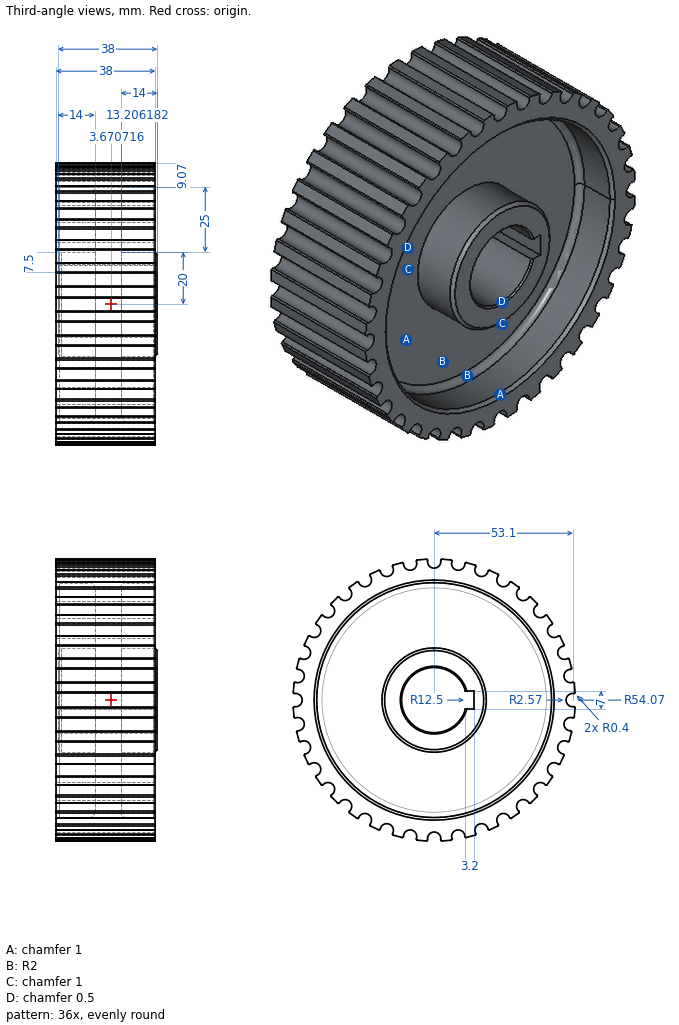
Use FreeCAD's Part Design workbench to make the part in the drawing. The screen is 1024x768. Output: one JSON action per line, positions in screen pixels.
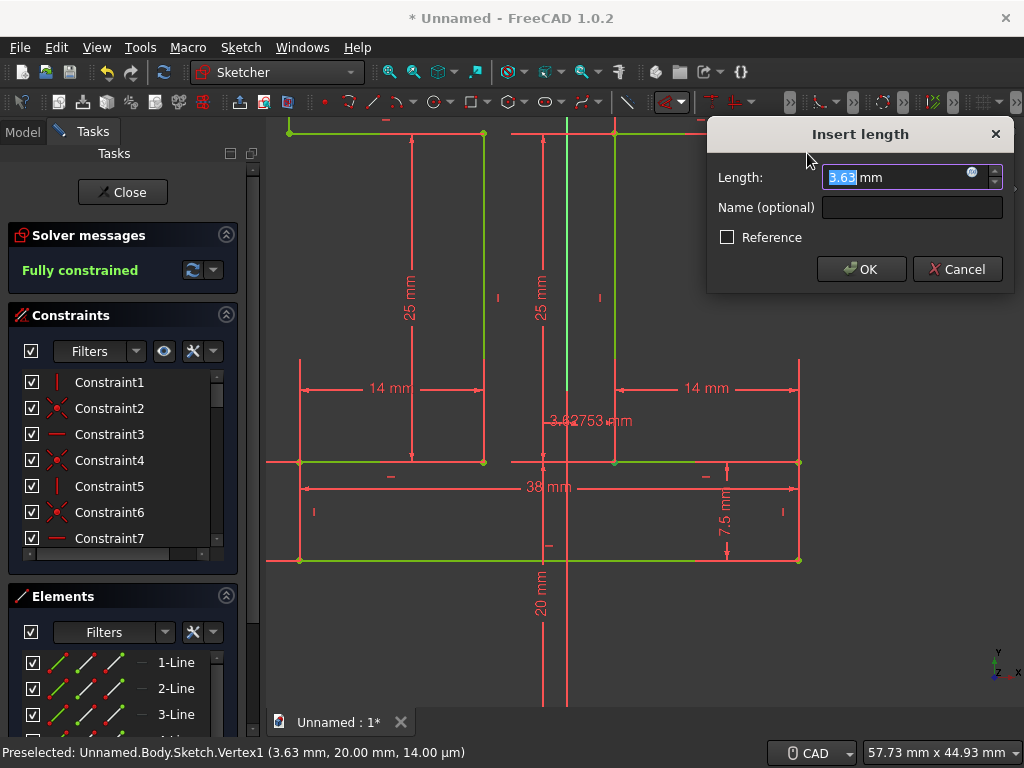
{"action": "type", "text": "3.670716"}
{"action": "key", "text": "Return"}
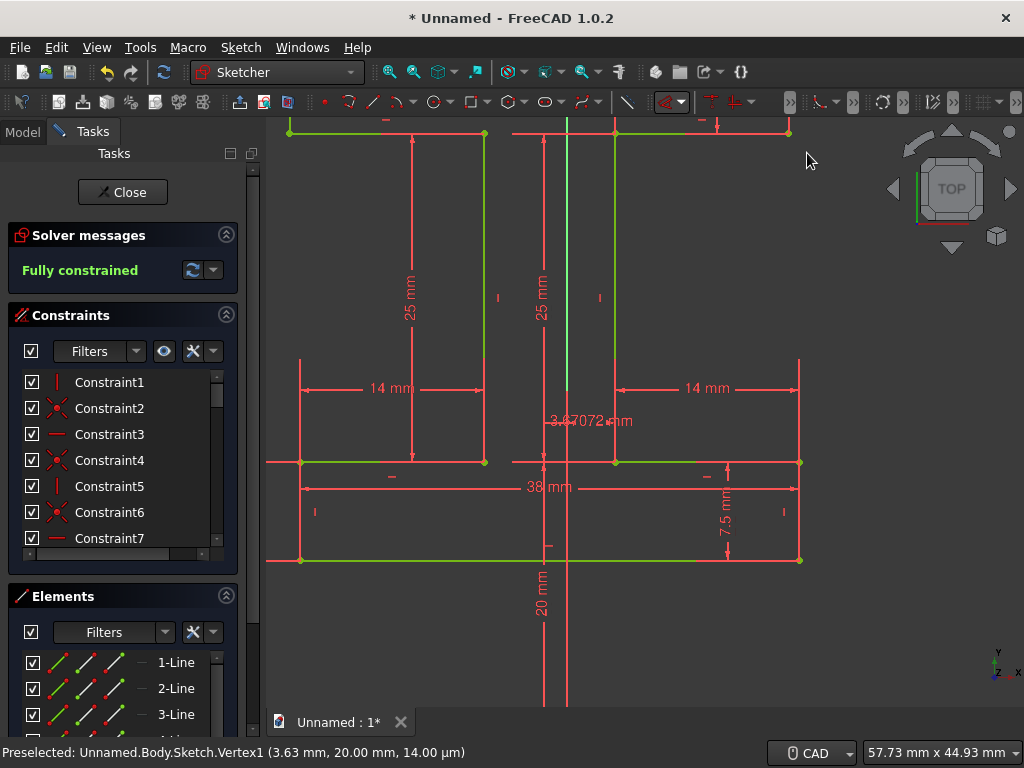
{"action": "left_click", "coordinate": [123, 192]}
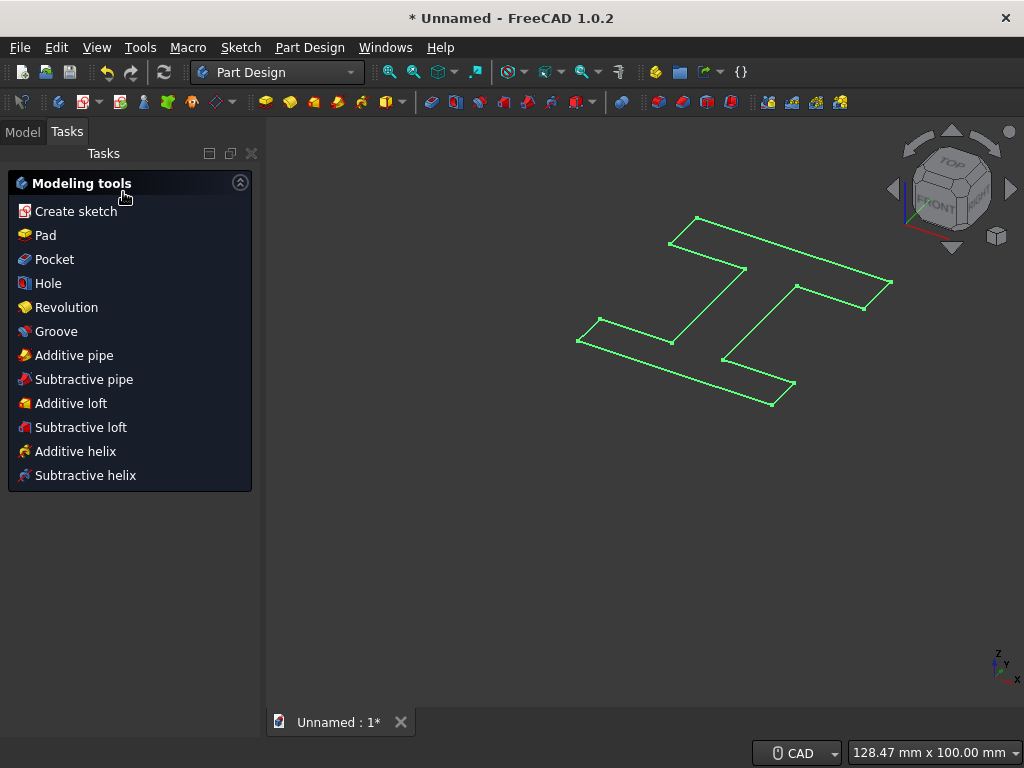
{"action": "left_click", "coordinate": [290, 102]}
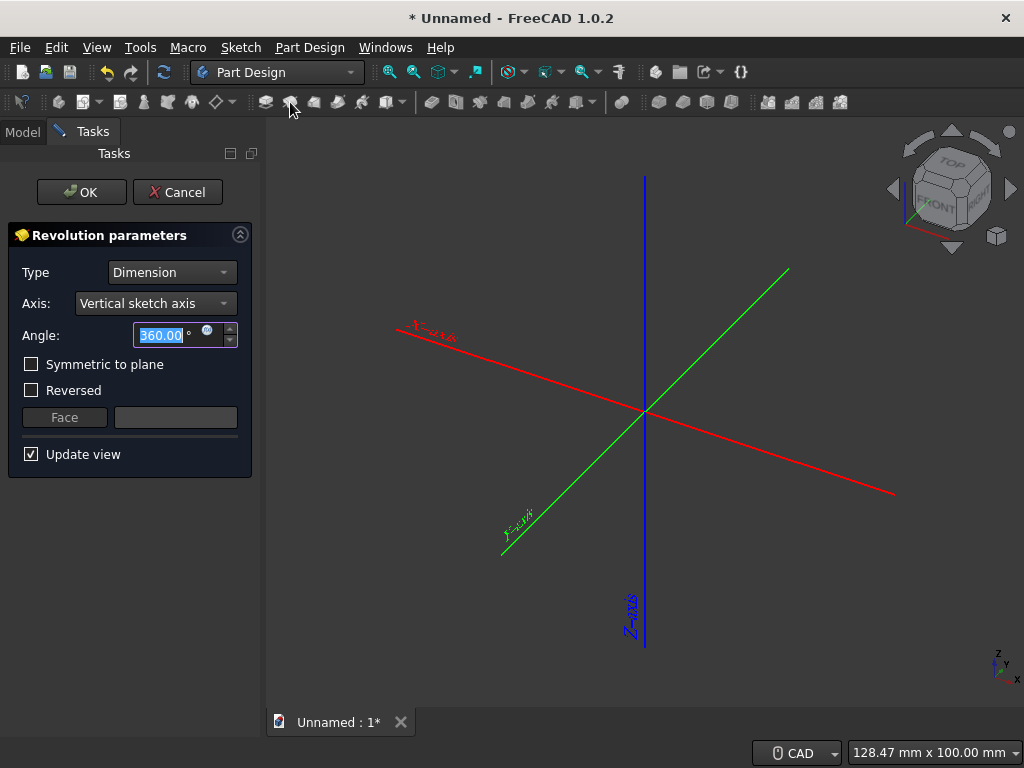
{"action": "left_click", "coordinate": [156, 304]}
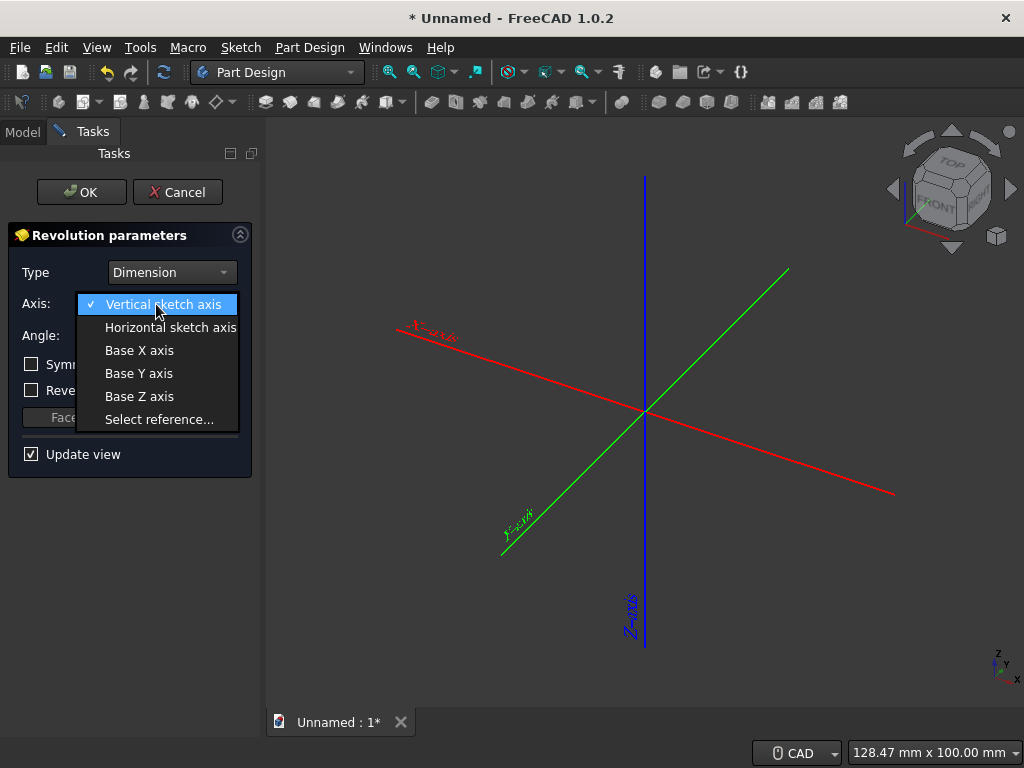
{"action": "left_click", "coordinate": [156, 328]}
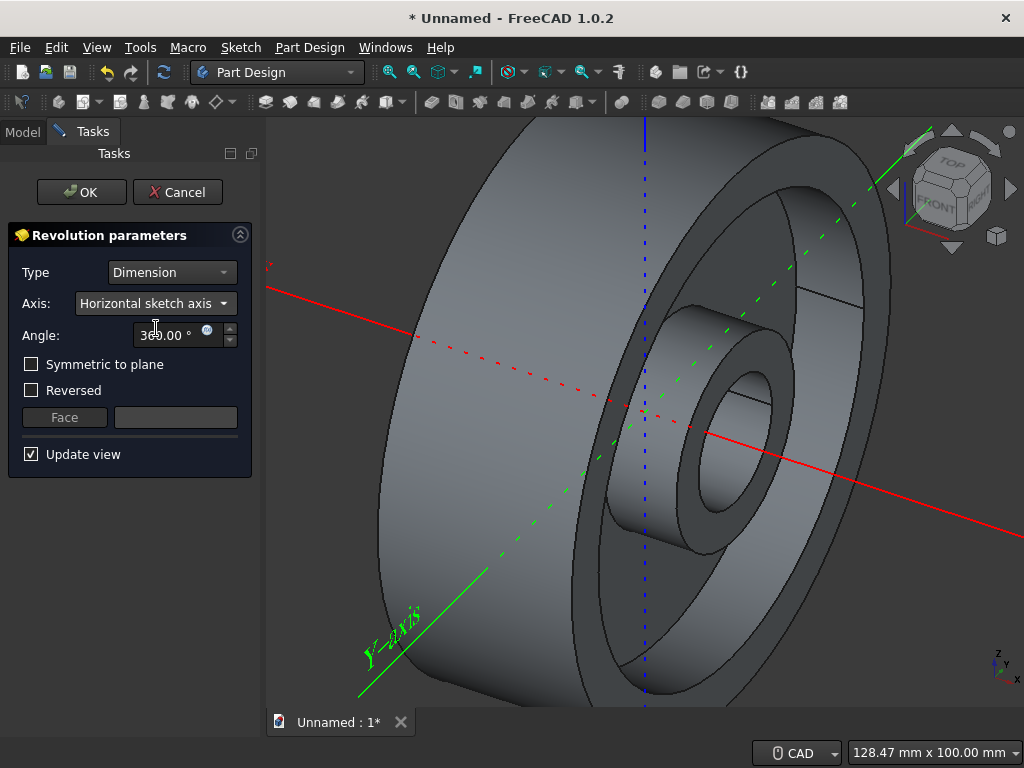
{"action": "left_click", "coordinate": [82, 192]}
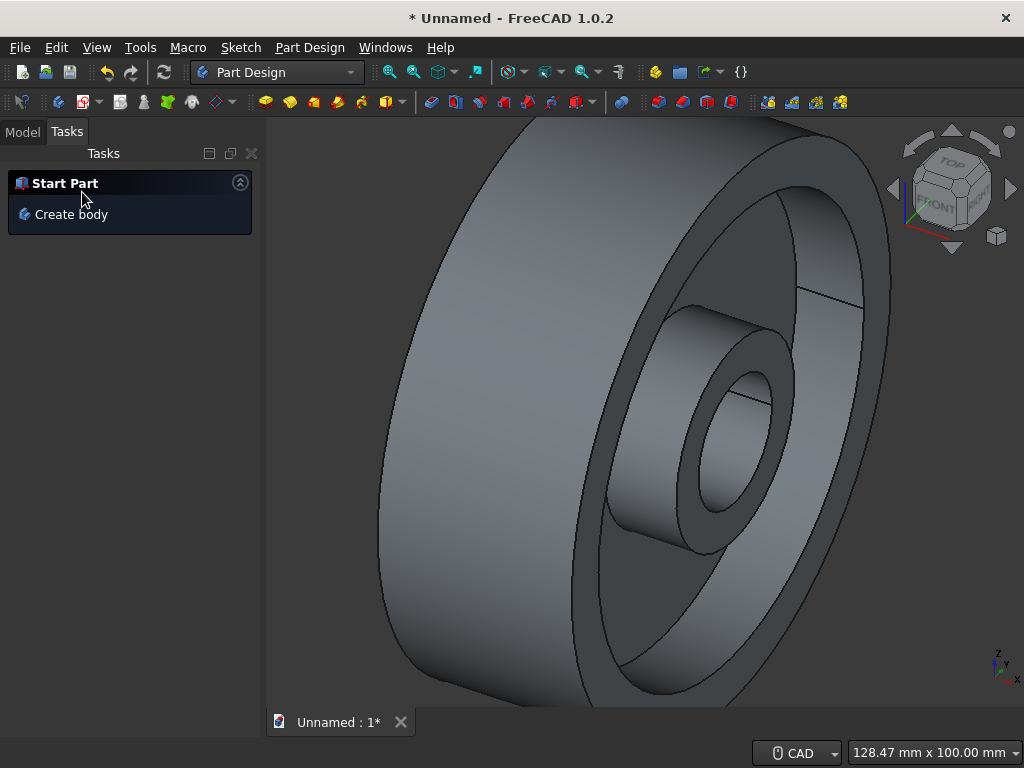
{"action": "left_click", "coordinate": [390, 72]}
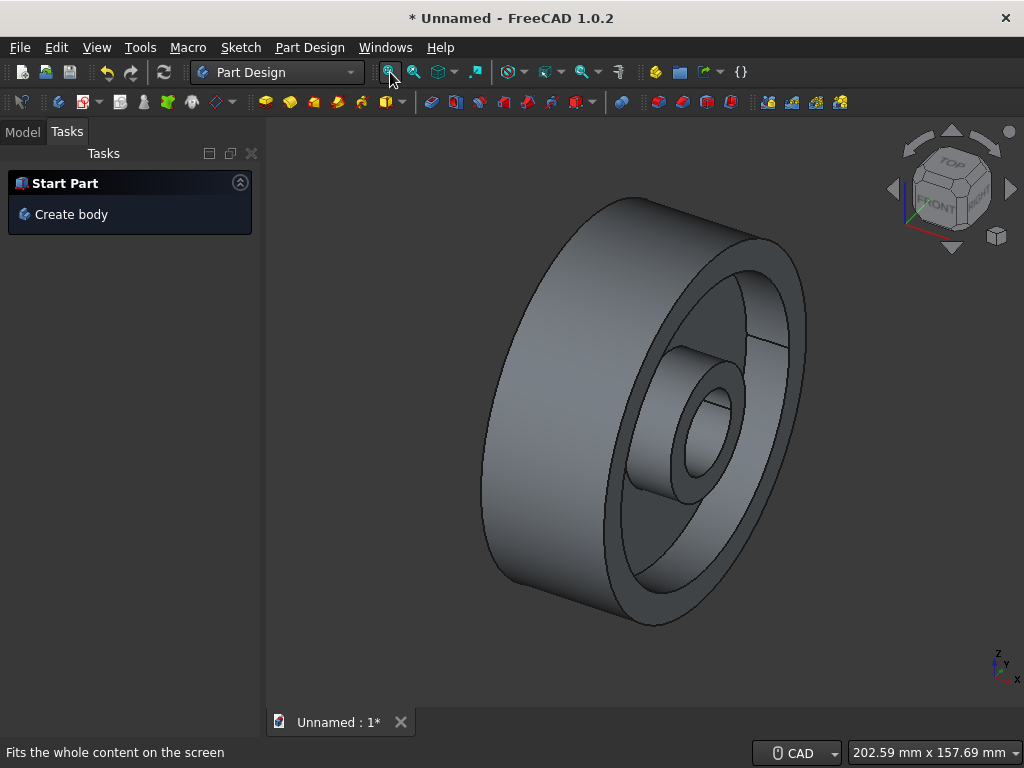
{"action": "left_click", "coordinate": [679, 588]}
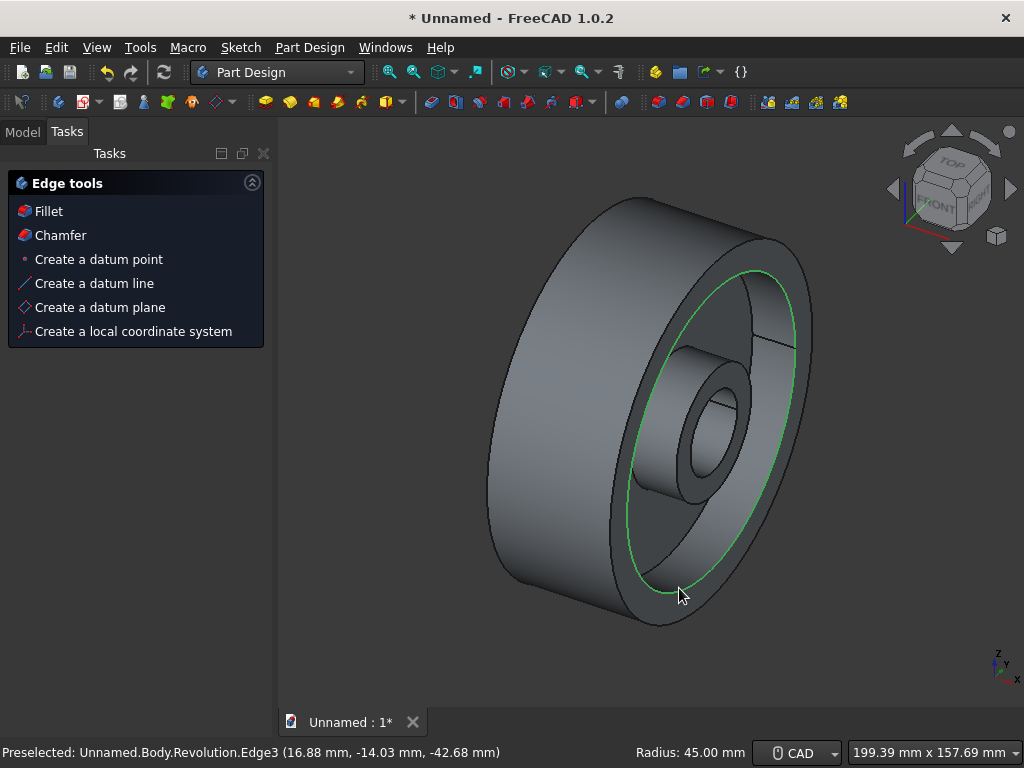
{"action": "key", "text": "0"}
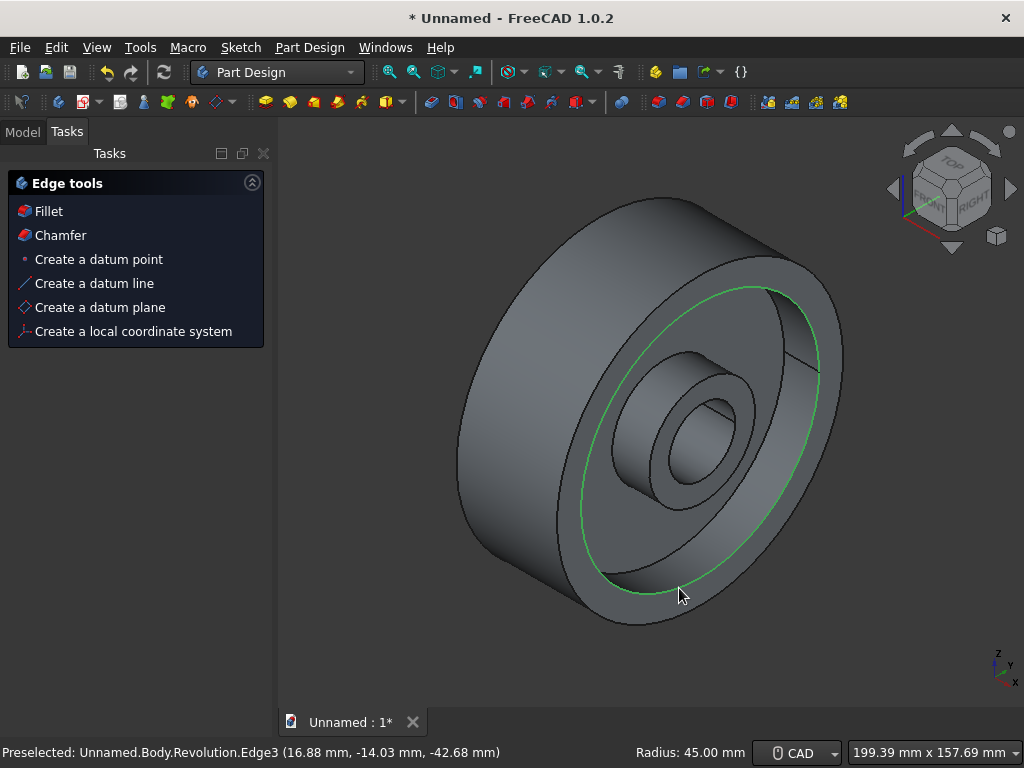
{"action": "key", "text": "2"}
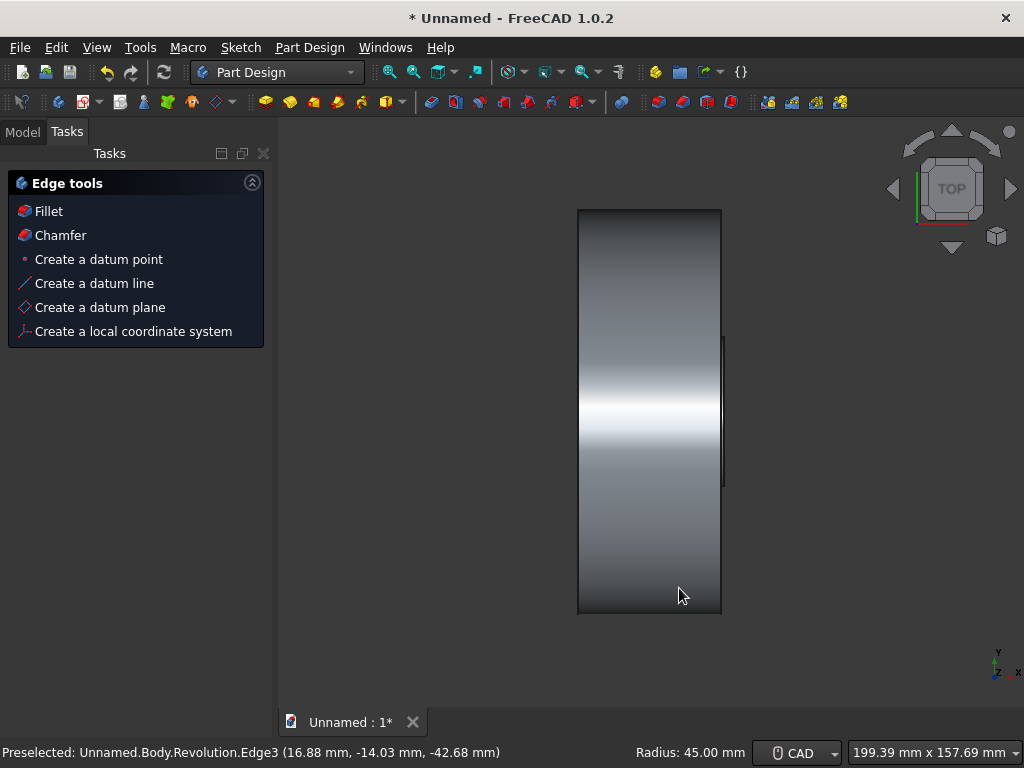
{"action": "key", "text": "1"}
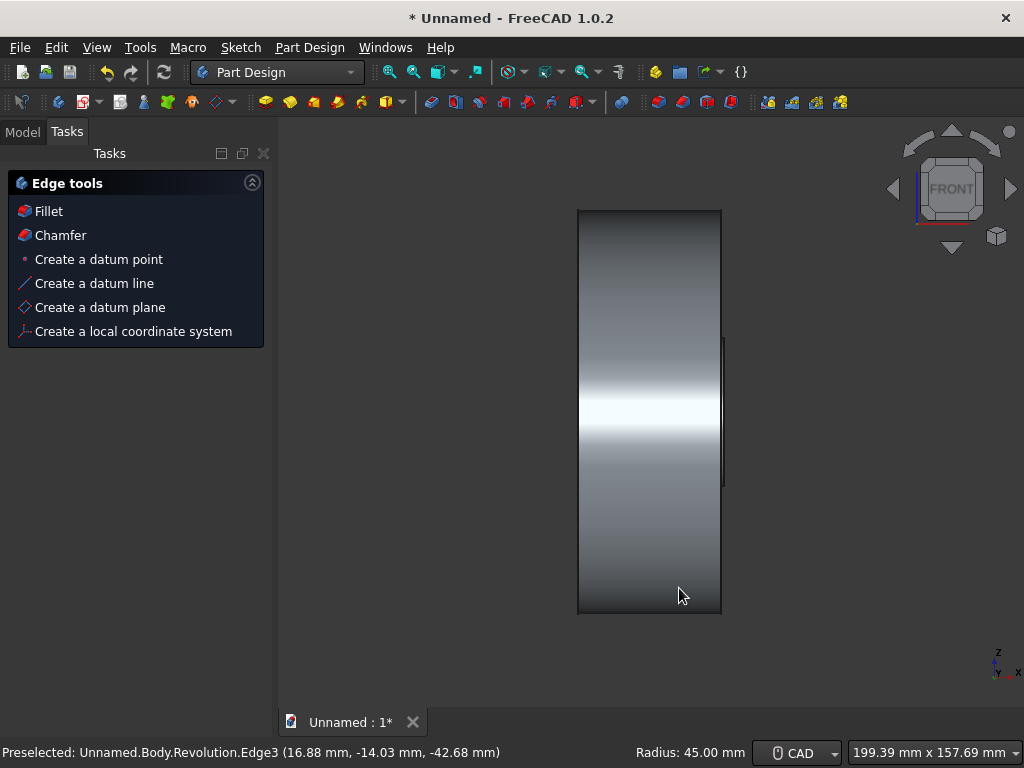
{"action": "key", "text": "3"}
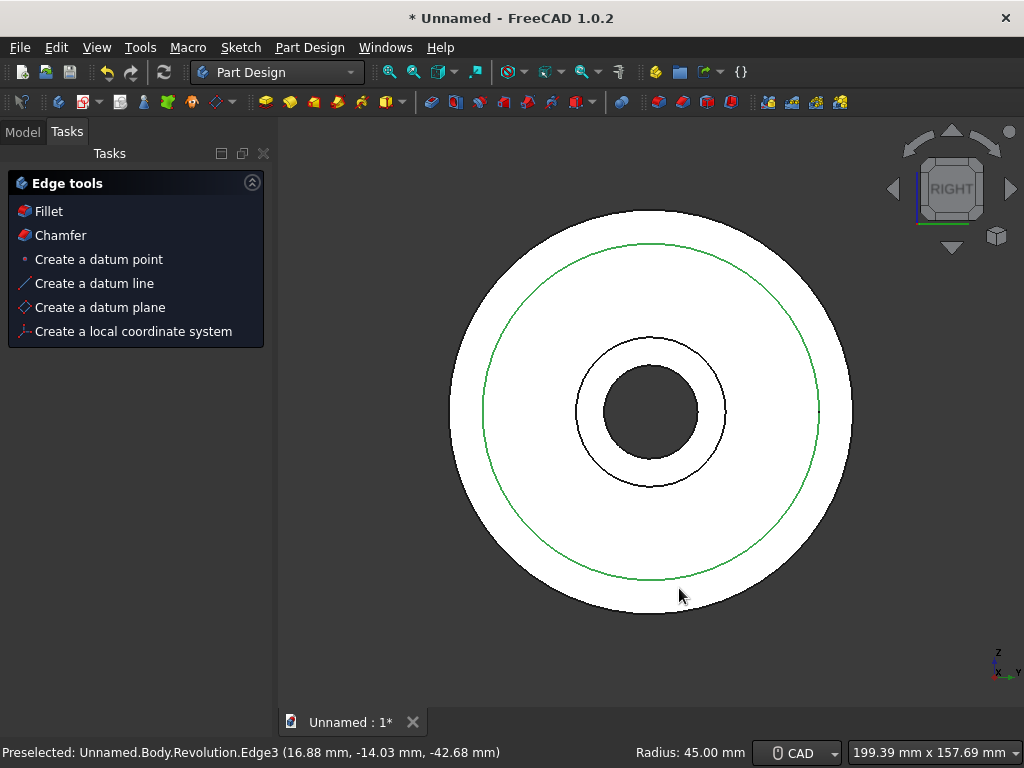
{"action": "key", "text": "5"}